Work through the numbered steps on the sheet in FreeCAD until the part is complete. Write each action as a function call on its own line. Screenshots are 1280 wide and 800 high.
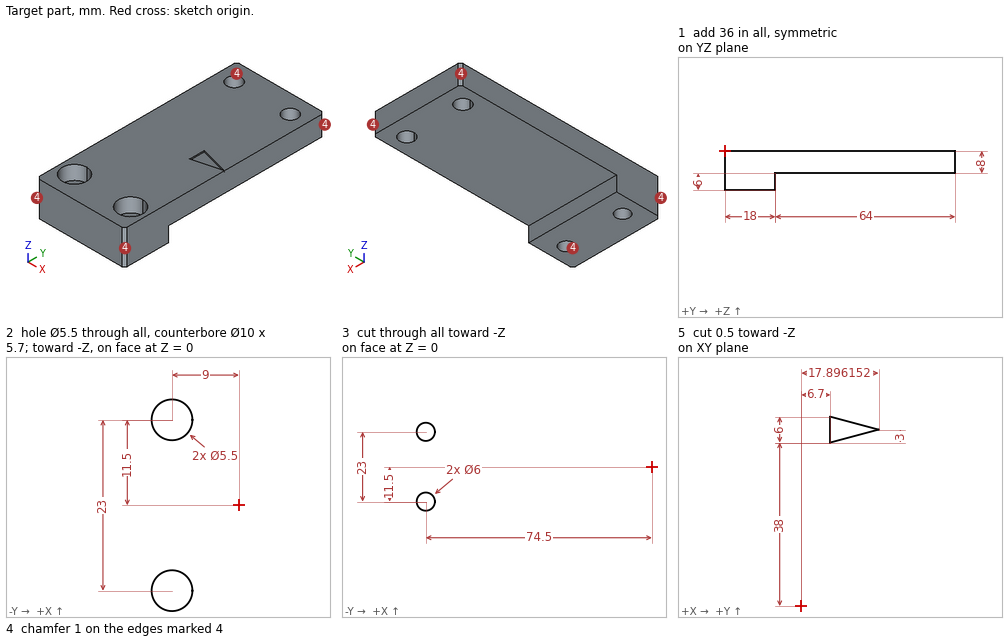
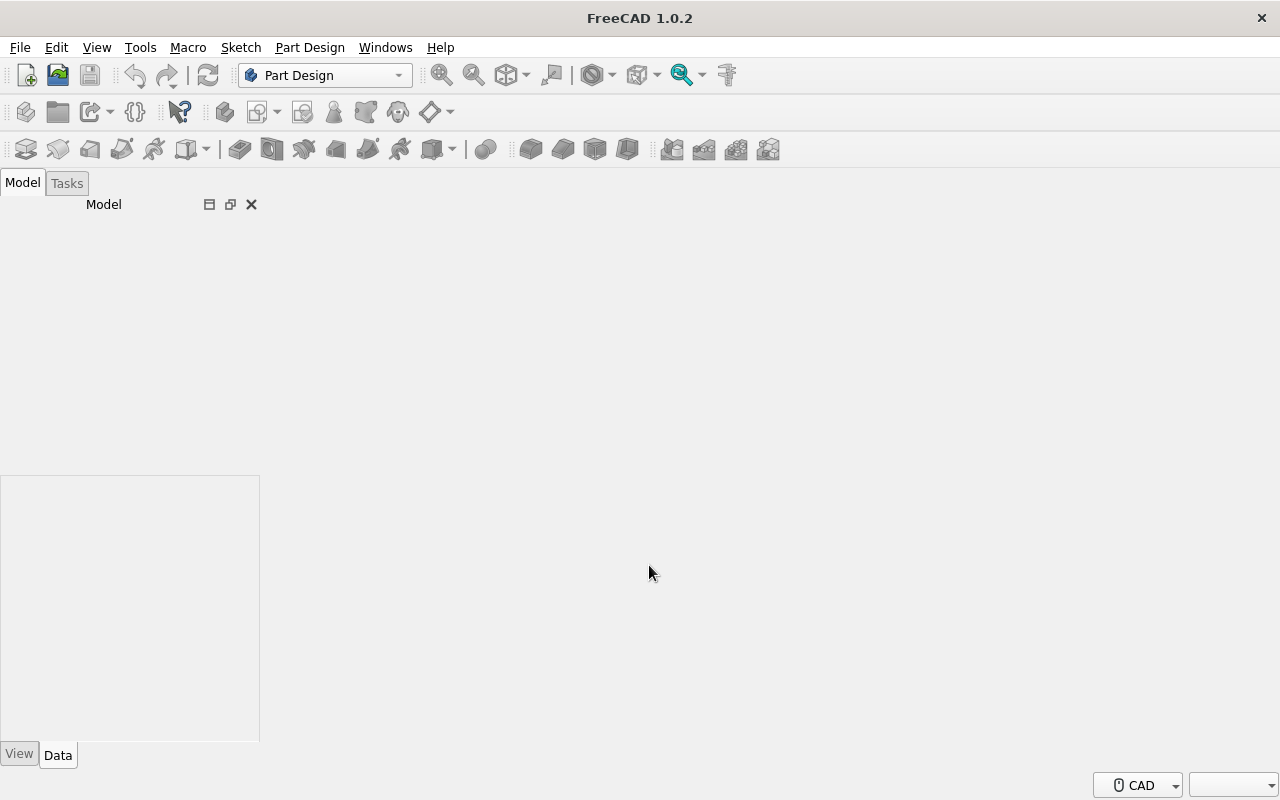
click(26, 76)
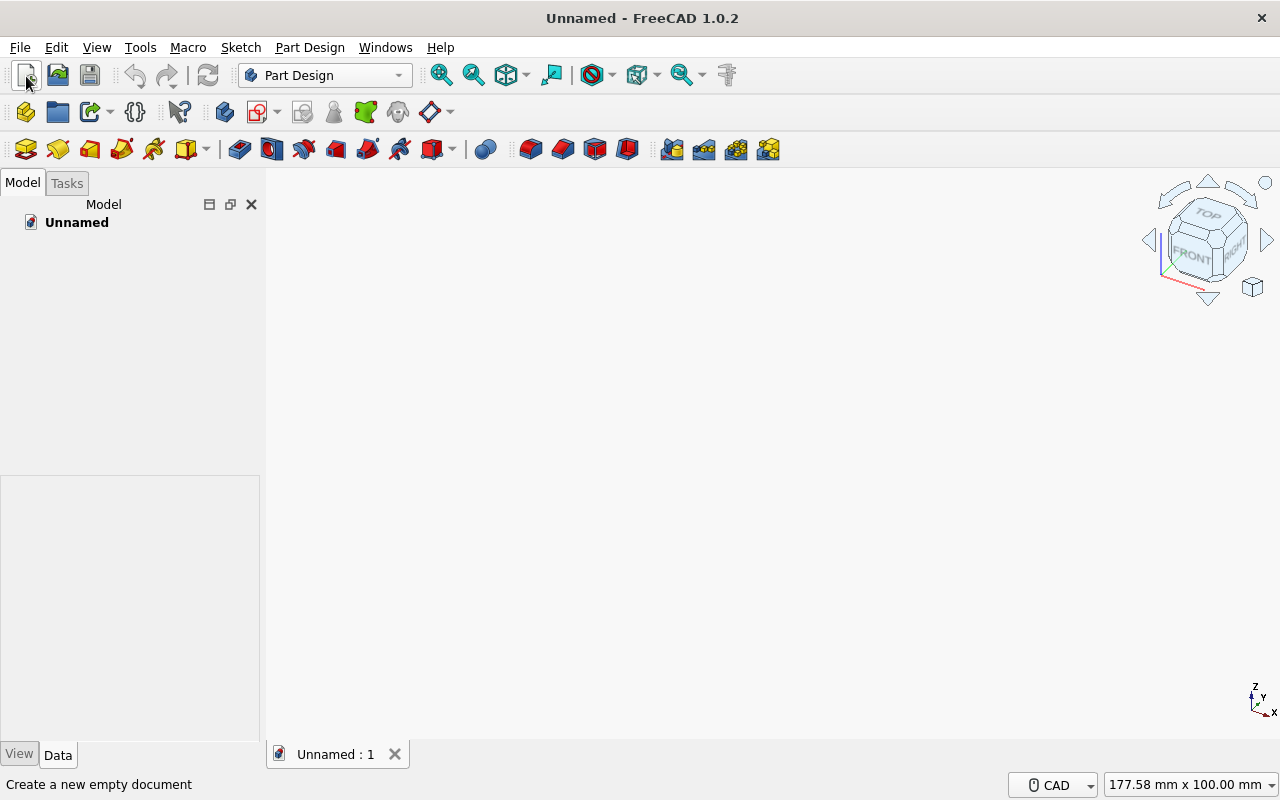
click(258, 112)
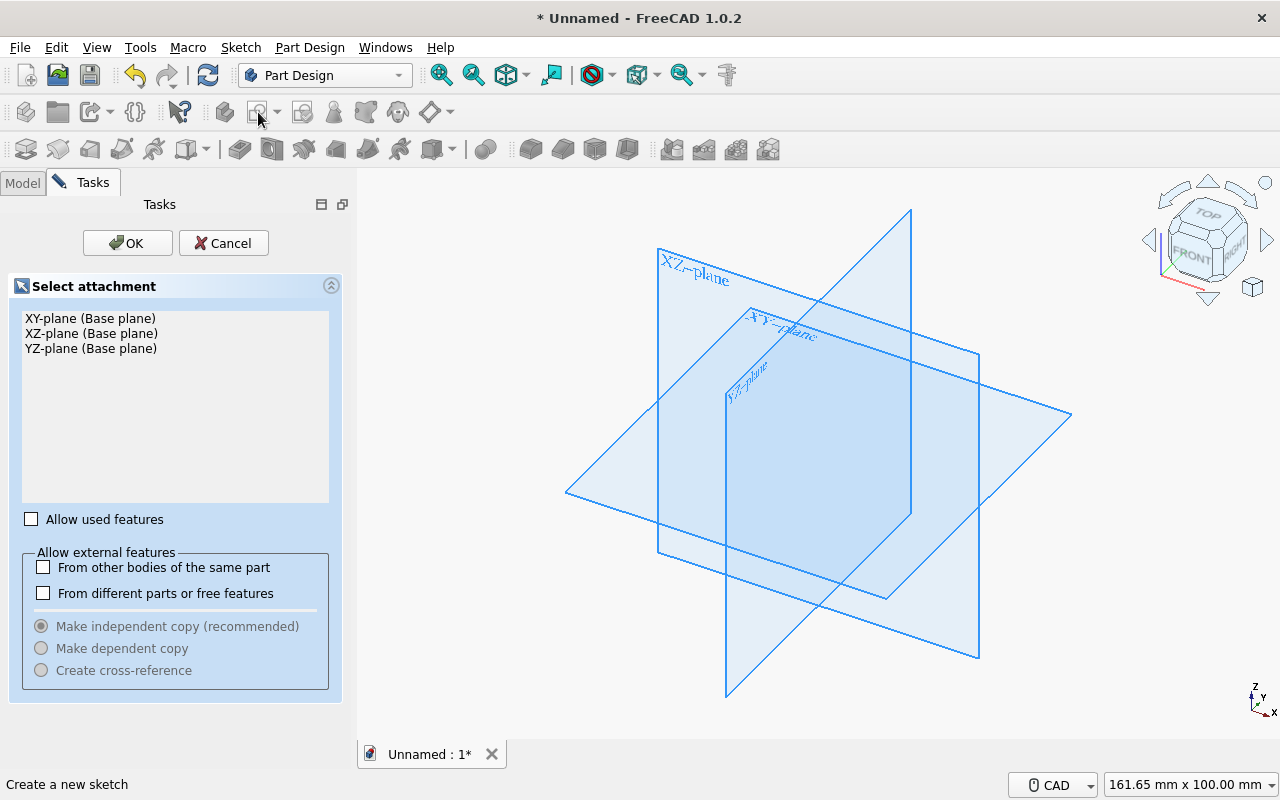
click(82, 348)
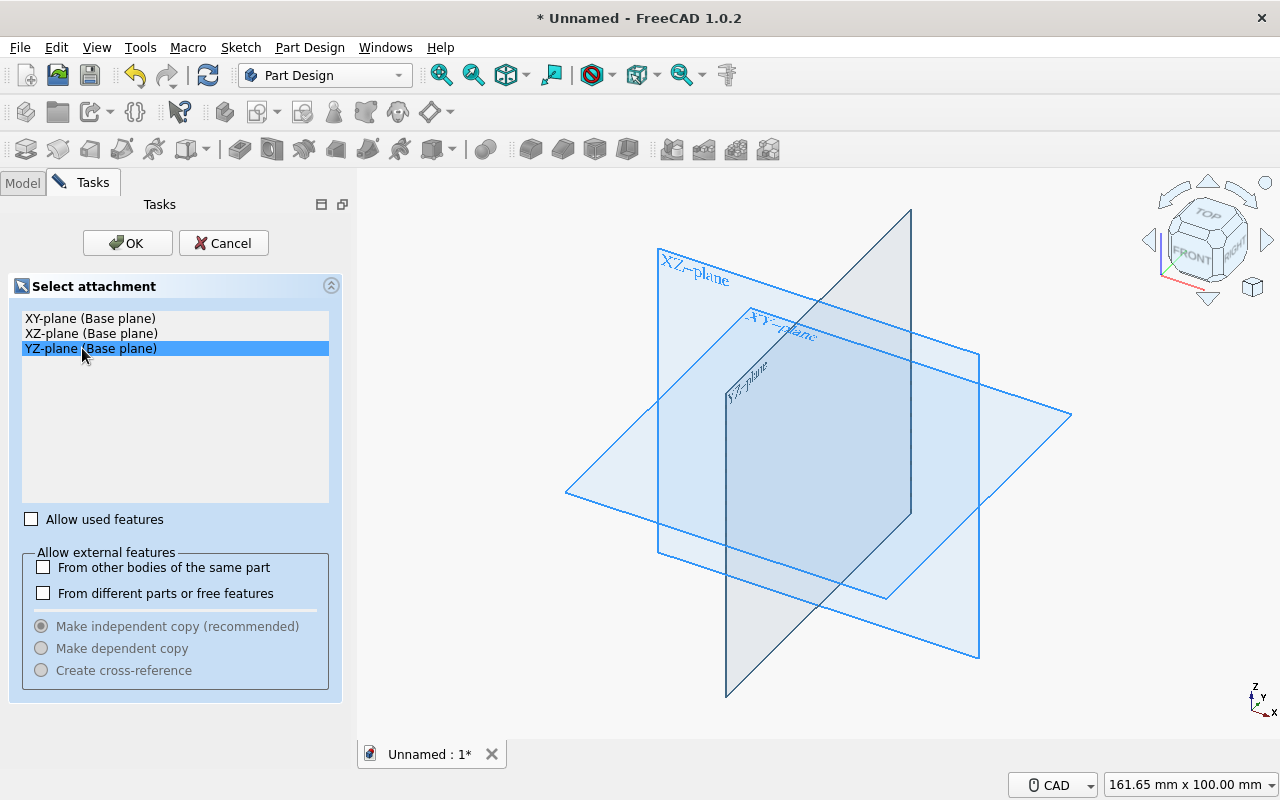
click(128, 243)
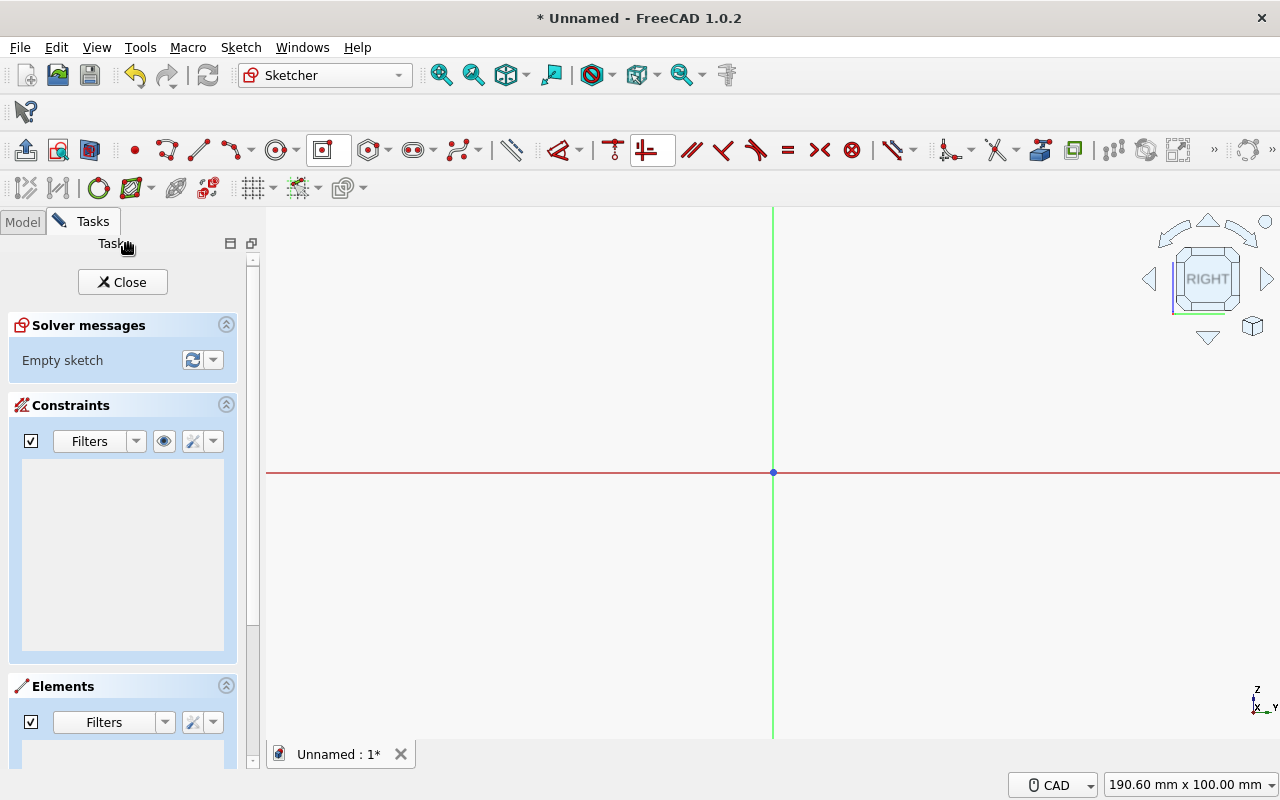
scroll(294, 305, down, 1)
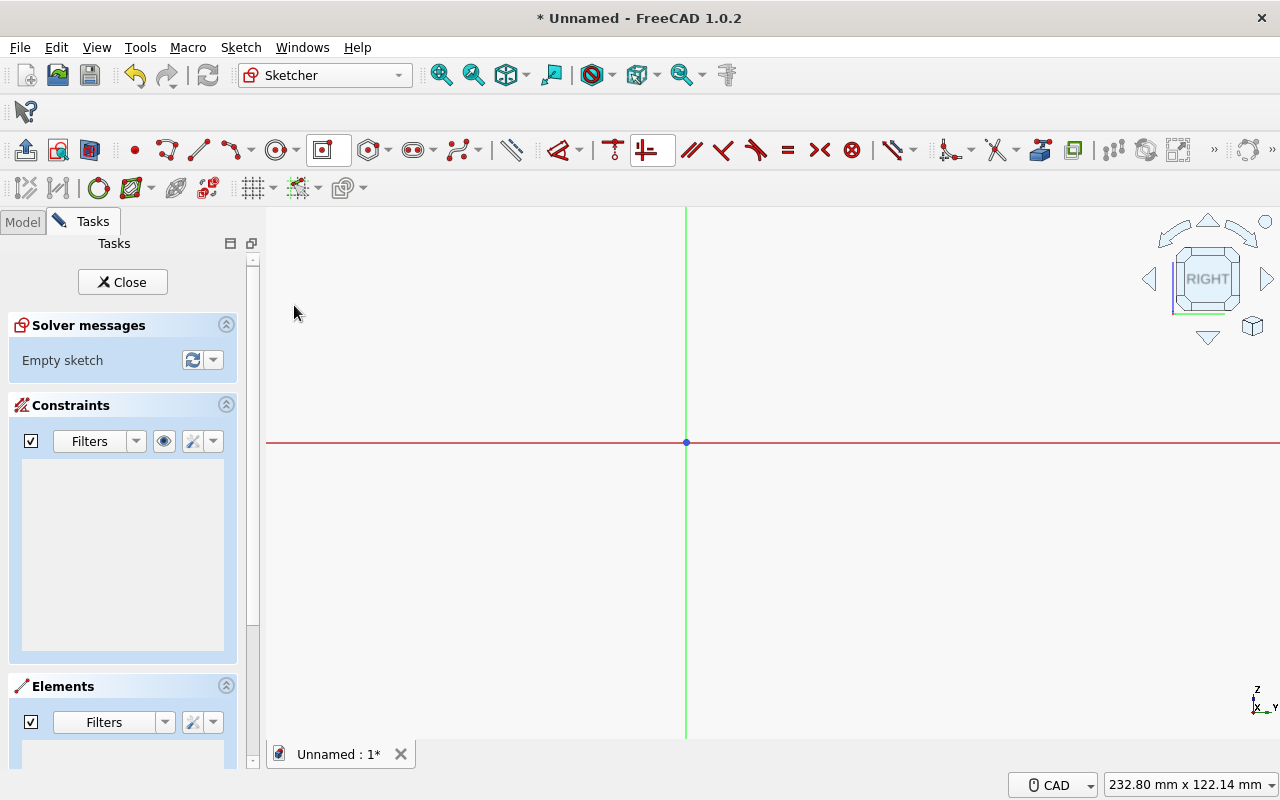
scroll(1115, 473, up, 2)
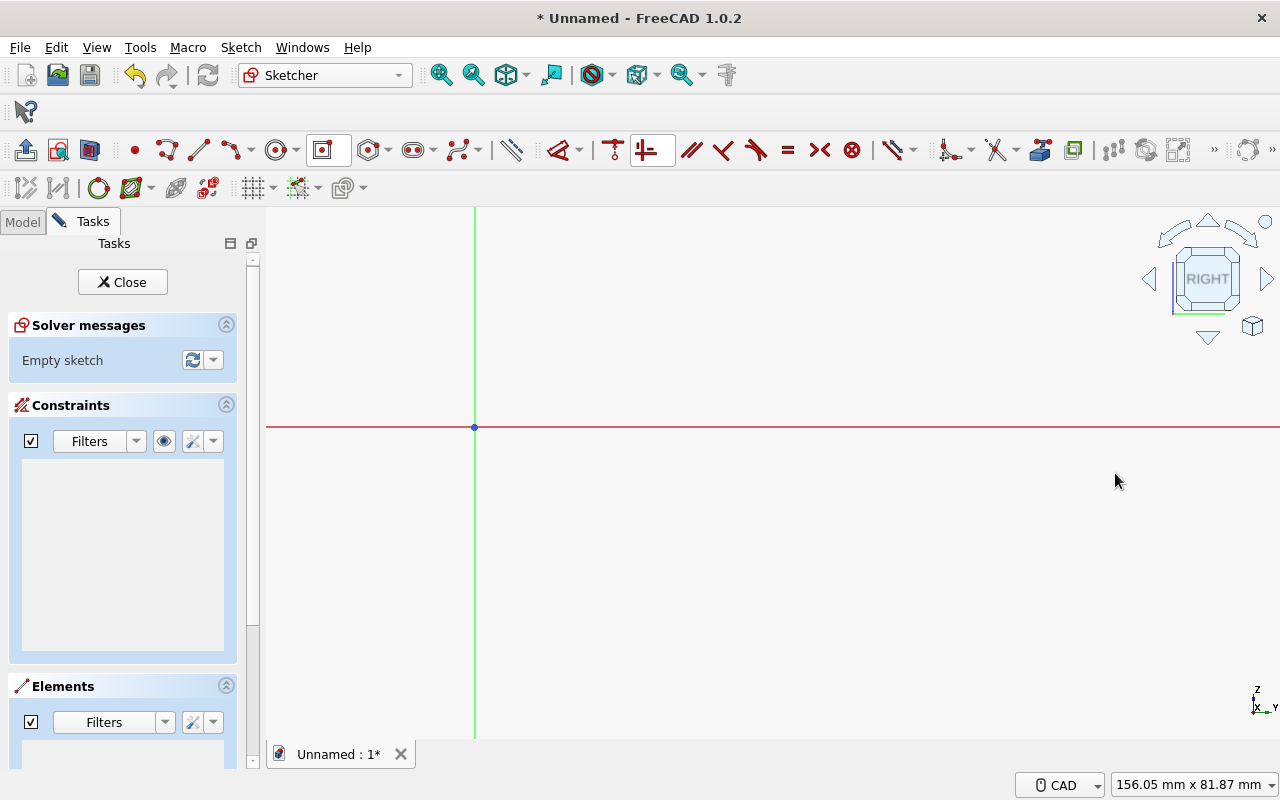
click(168, 150)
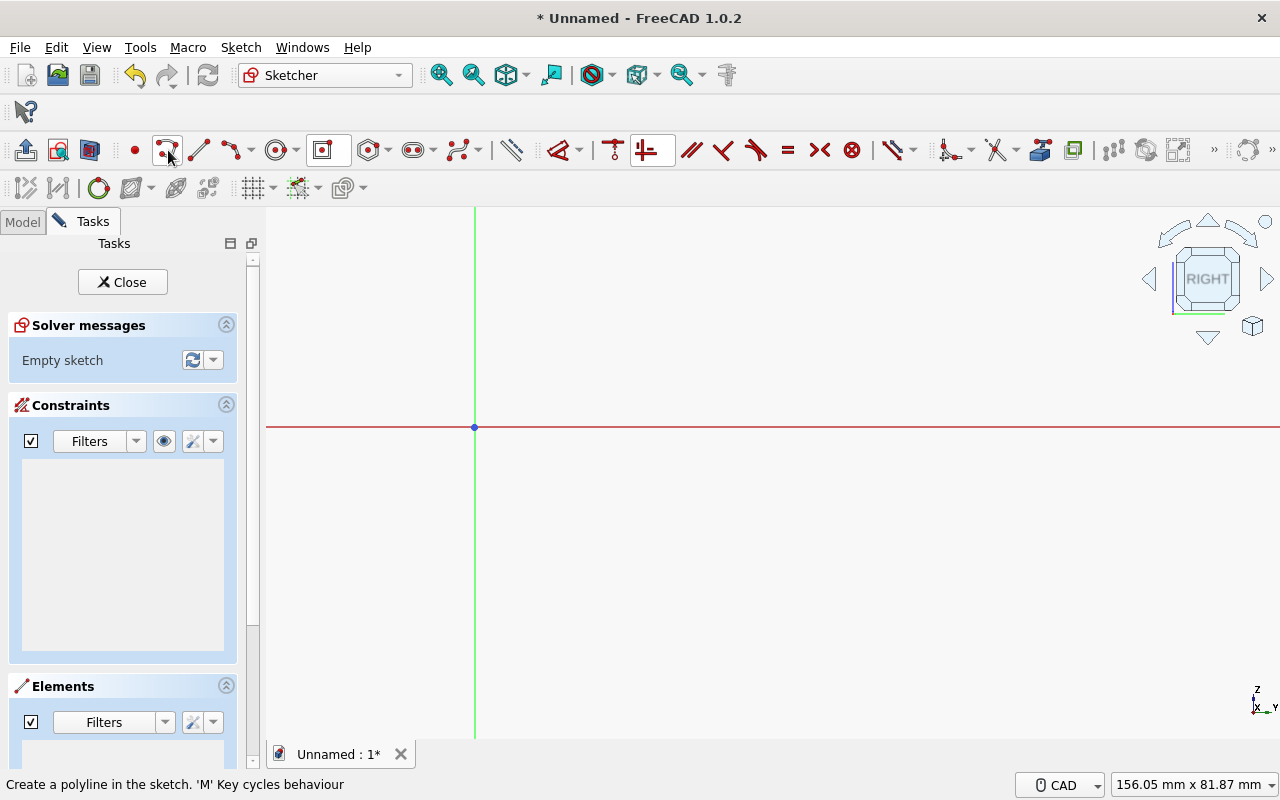
click(475, 427)
click(484, 518)
click(592, 518)
click(592, 479)
click(1008, 479)
click(1008, 436)
click(475, 427)
key(Escape)
key(Escape)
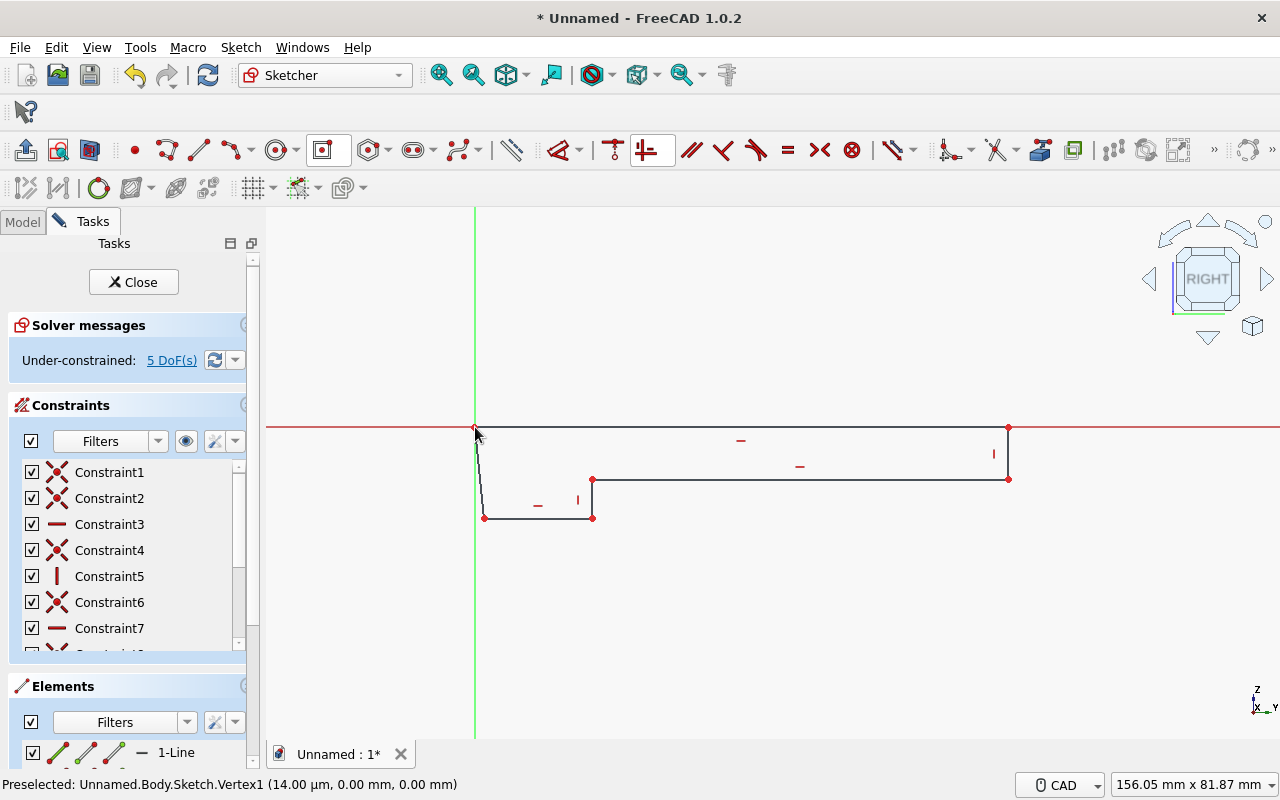
click(478, 455)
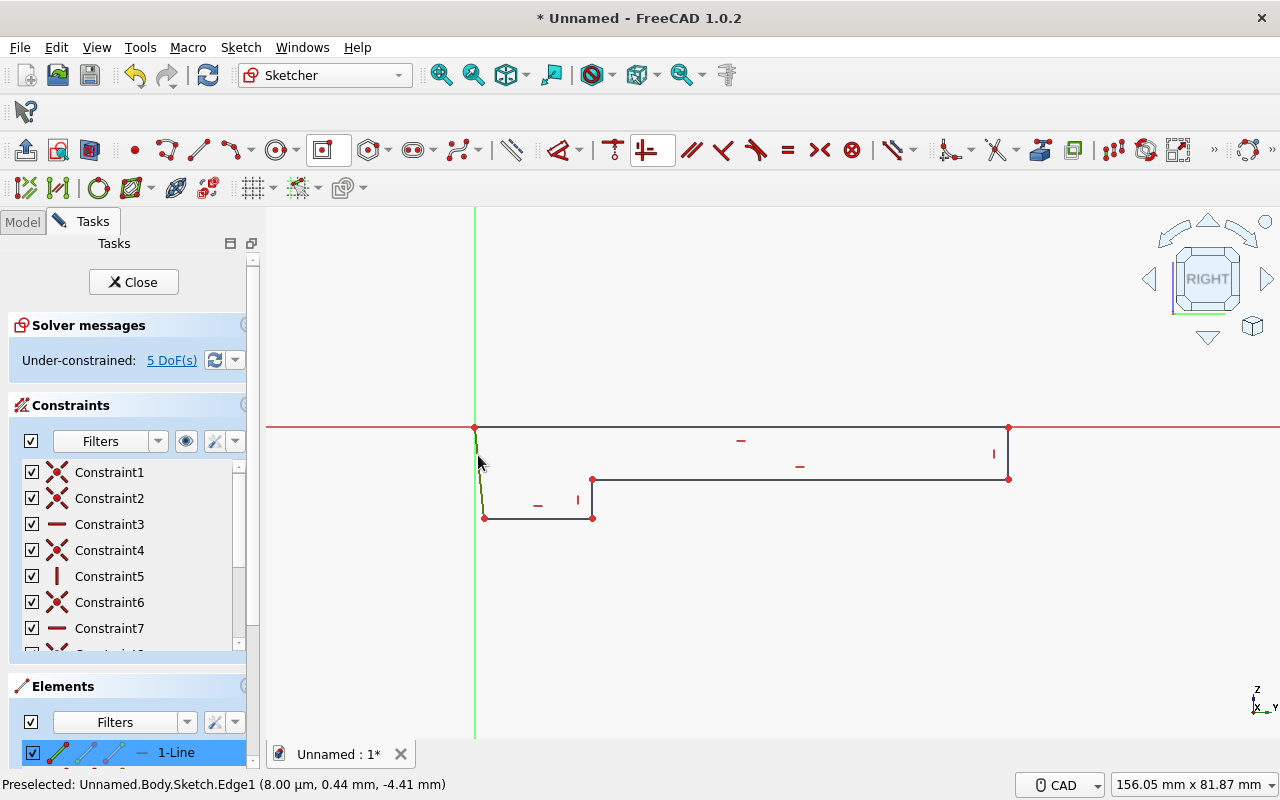
click(670, 150)